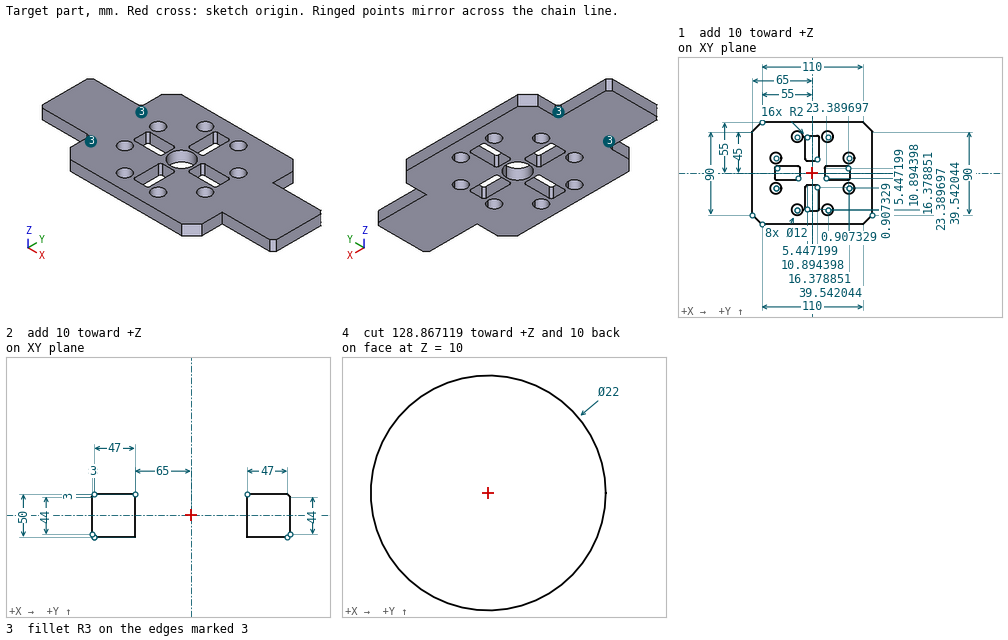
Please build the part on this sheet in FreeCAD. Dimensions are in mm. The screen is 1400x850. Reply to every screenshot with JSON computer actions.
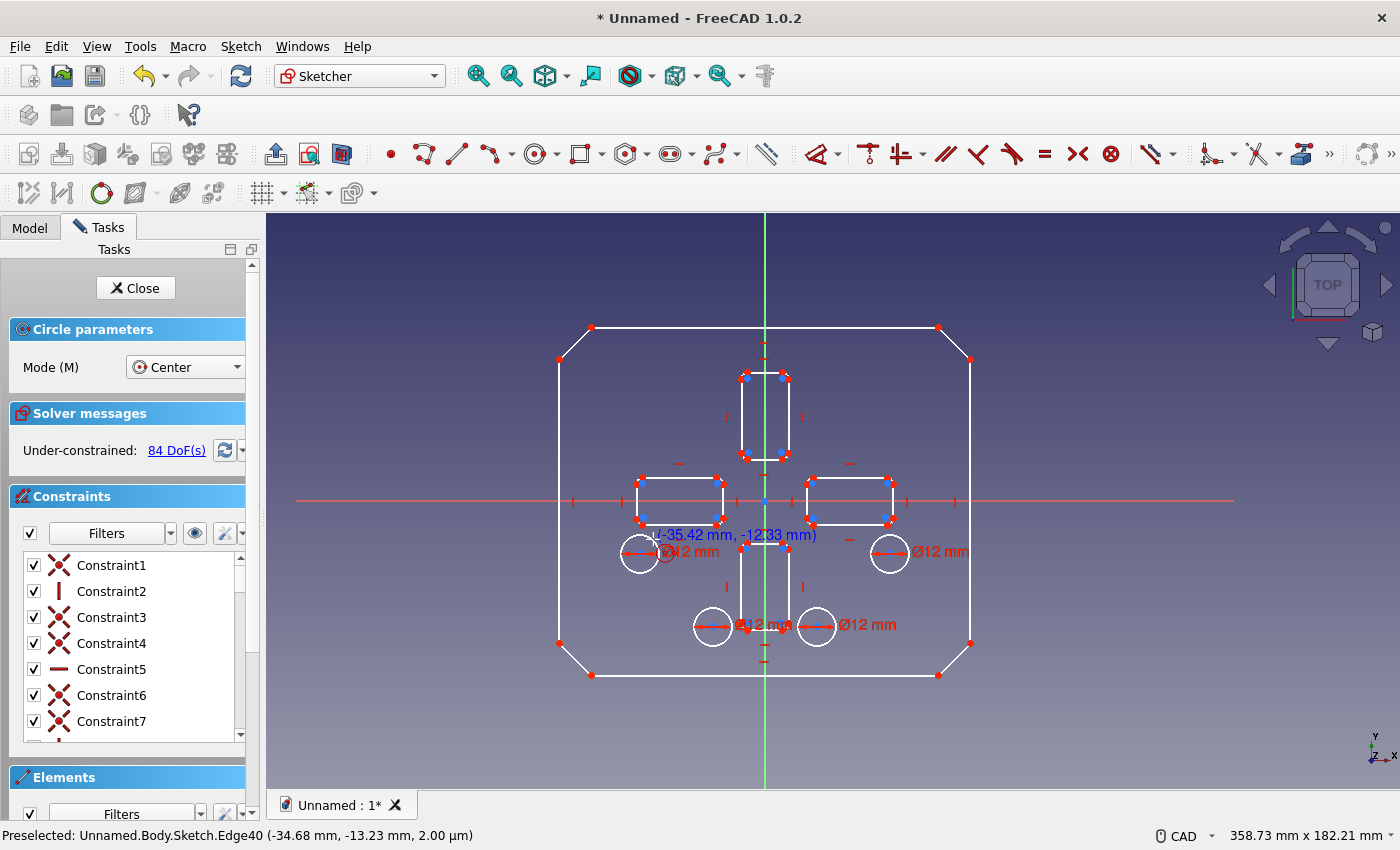
{"action": "left_click", "coordinate": [890, 449]}
{"action": "mouse_move", "coordinate": [903, 436]}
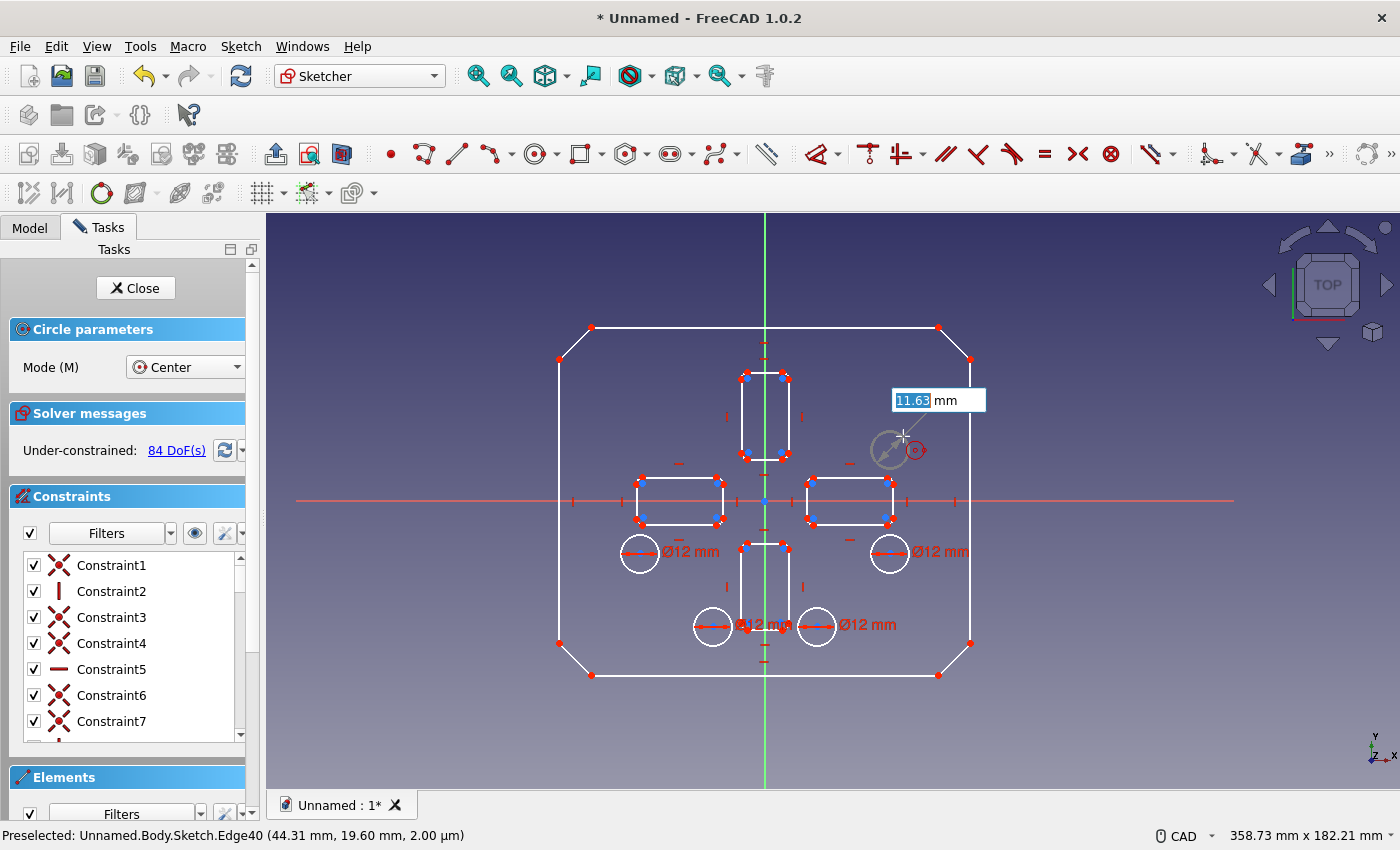
{"action": "type", "text": "12"}
{"action": "key", "text": "Return"}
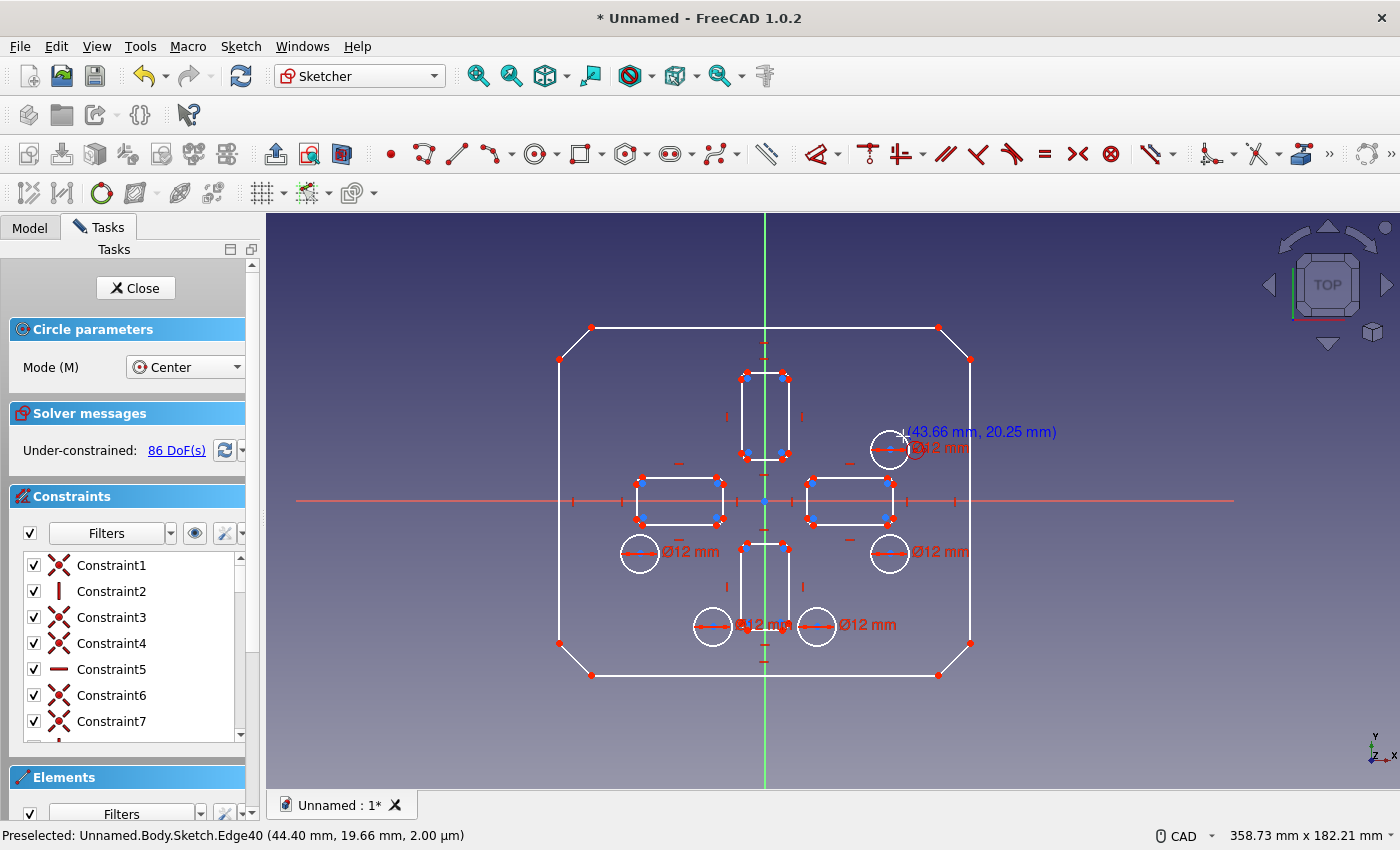
{"action": "left_click", "coordinate": [817, 376]}
{"action": "mouse_move", "coordinate": [830, 363]}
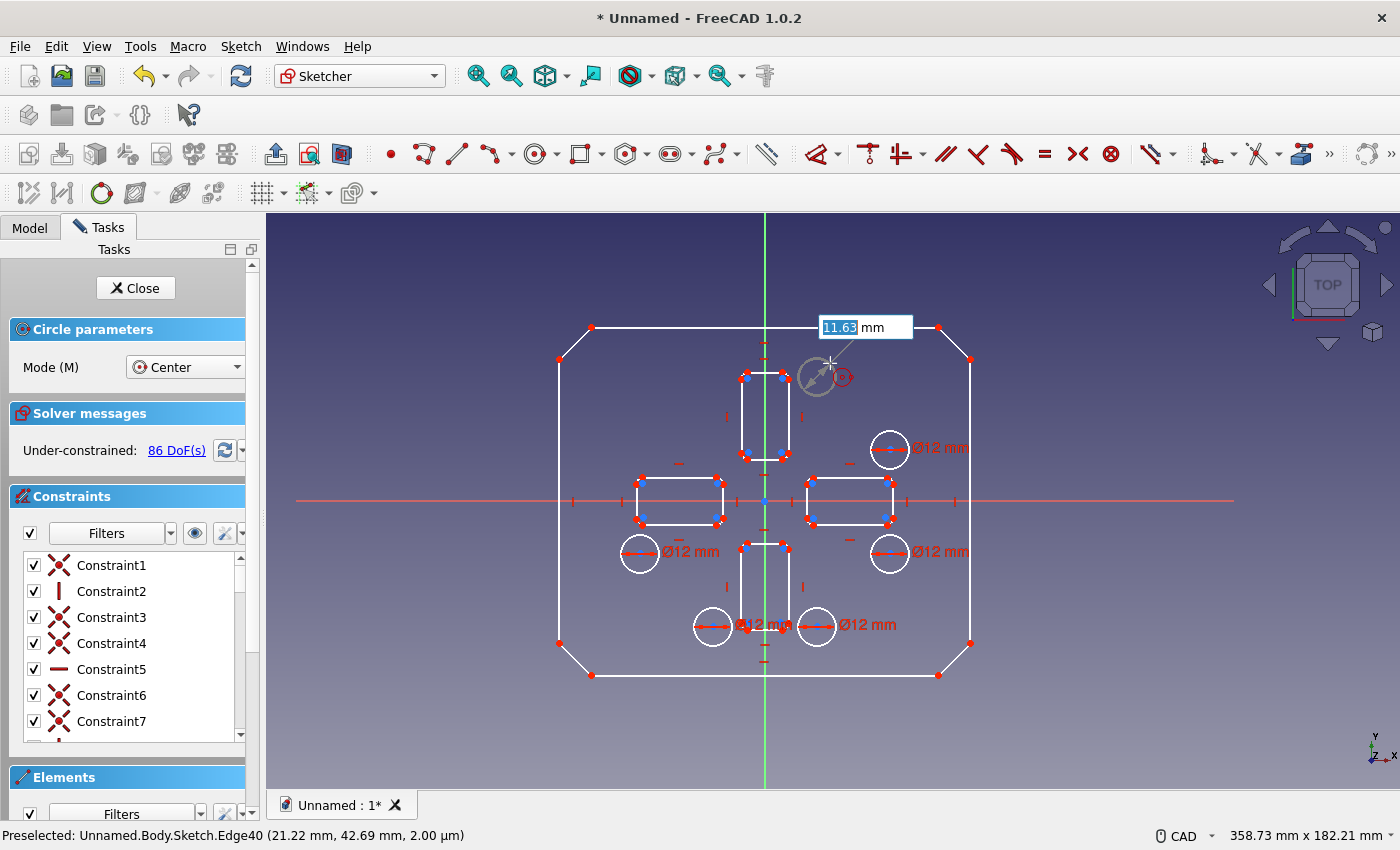
{"action": "type", "text": "12"}
{"action": "key", "text": "Return"}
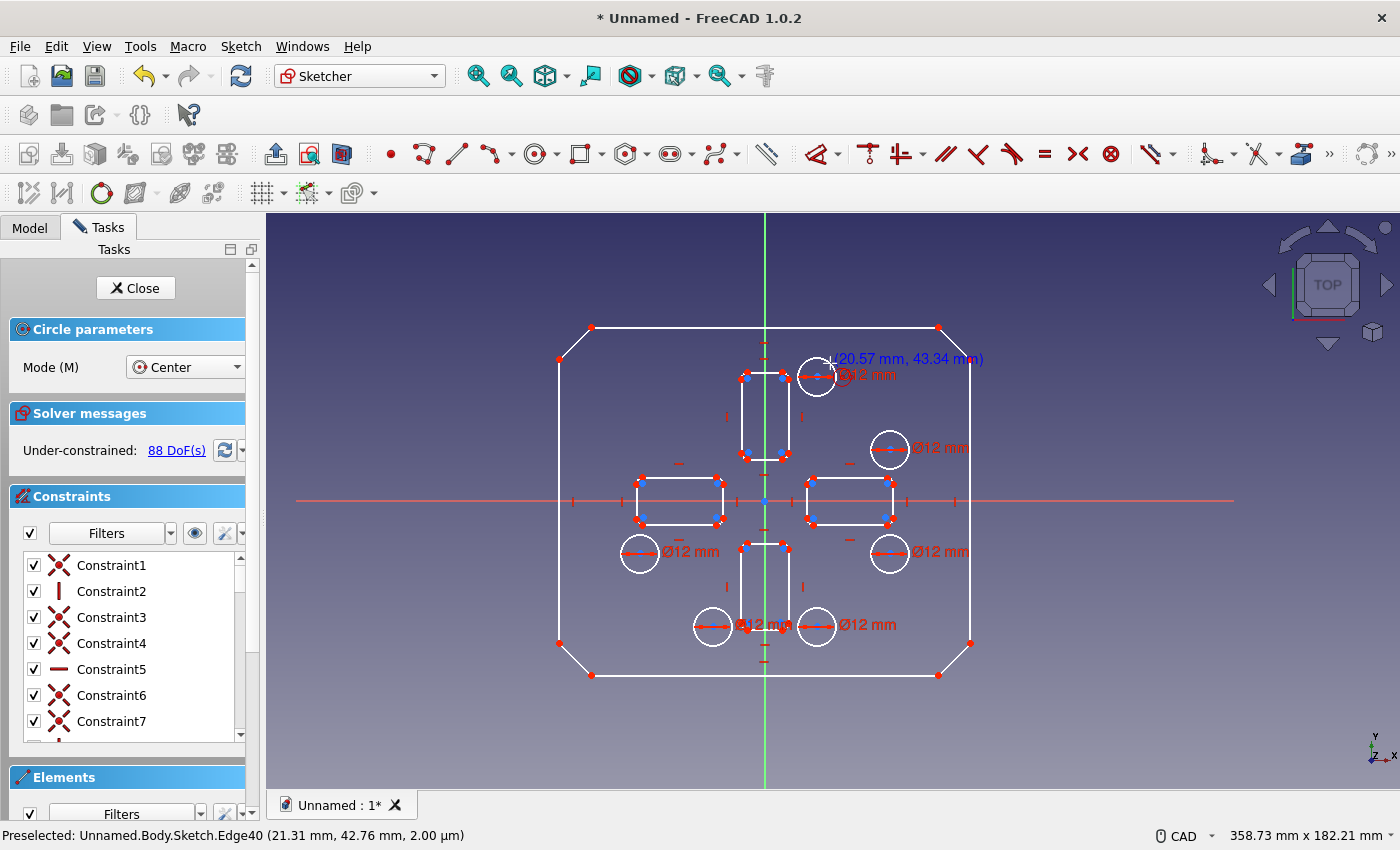
{"action": "left_click", "coordinate": [640, 449]}
{"action": "mouse_move", "coordinate": [653, 436]}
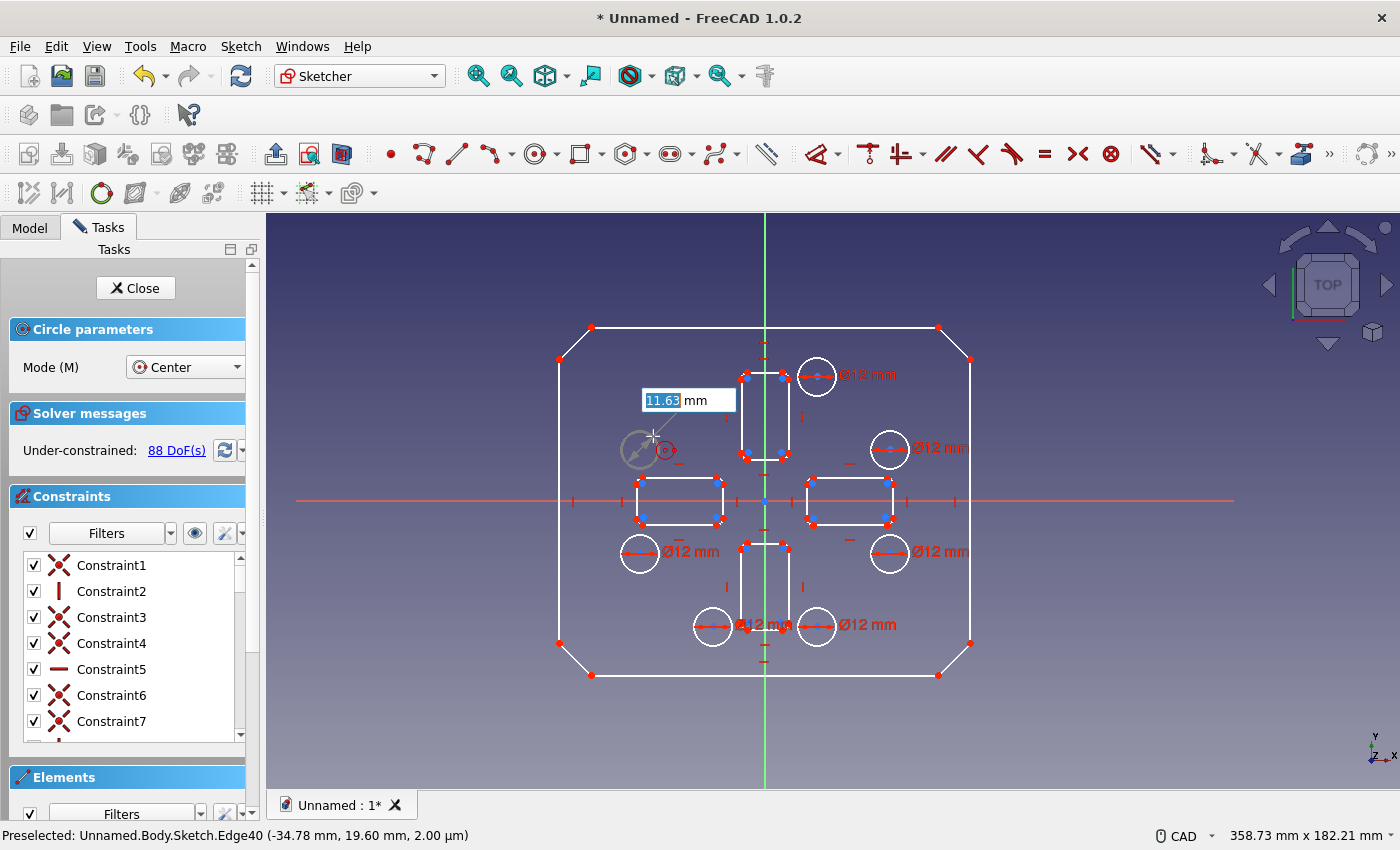
{"action": "type", "text": "12"}
{"action": "key", "text": "Return"}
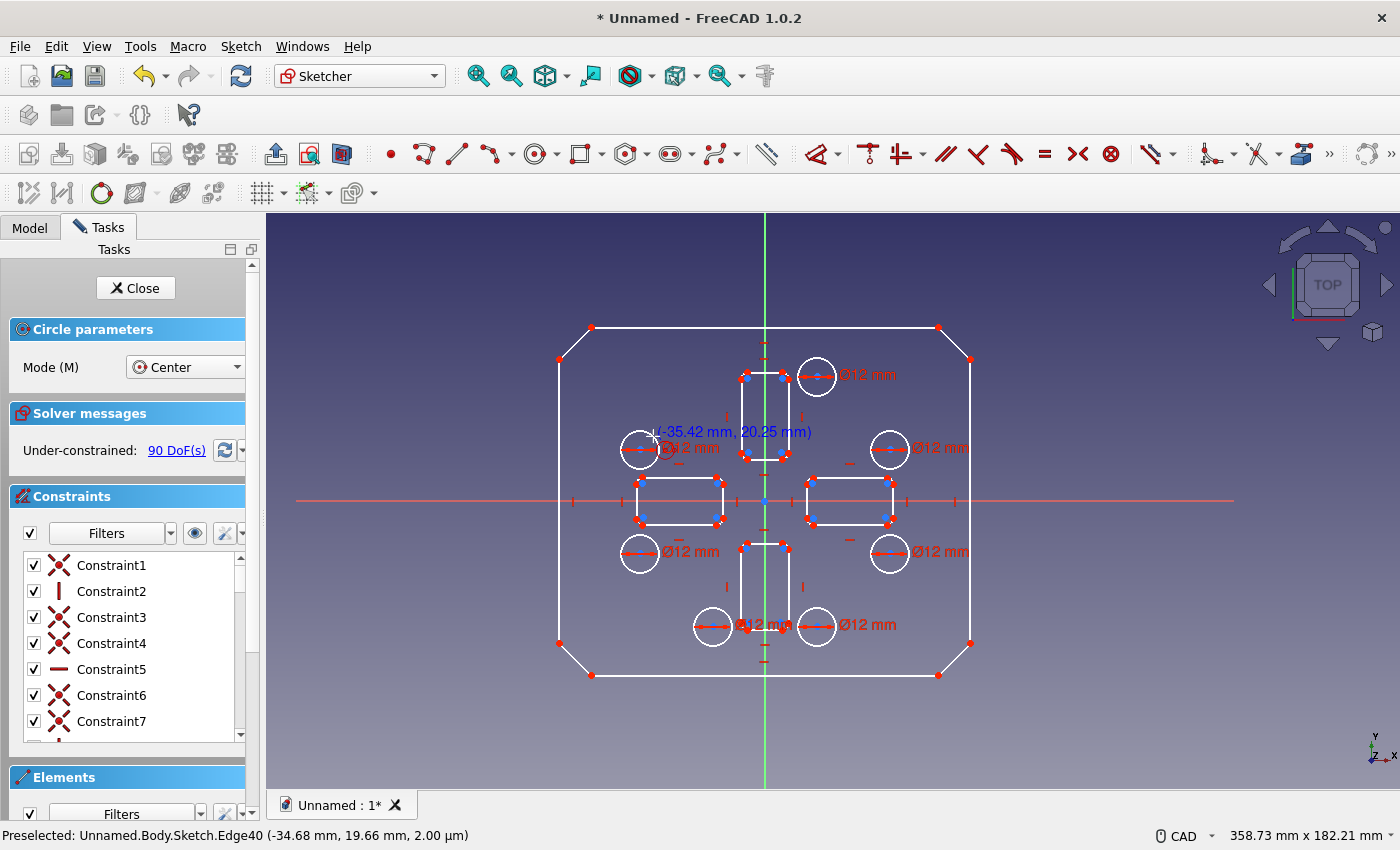
{"action": "left_click", "coordinate": [713, 376]}
{"action": "mouse_move", "coordinate": [727, 363]}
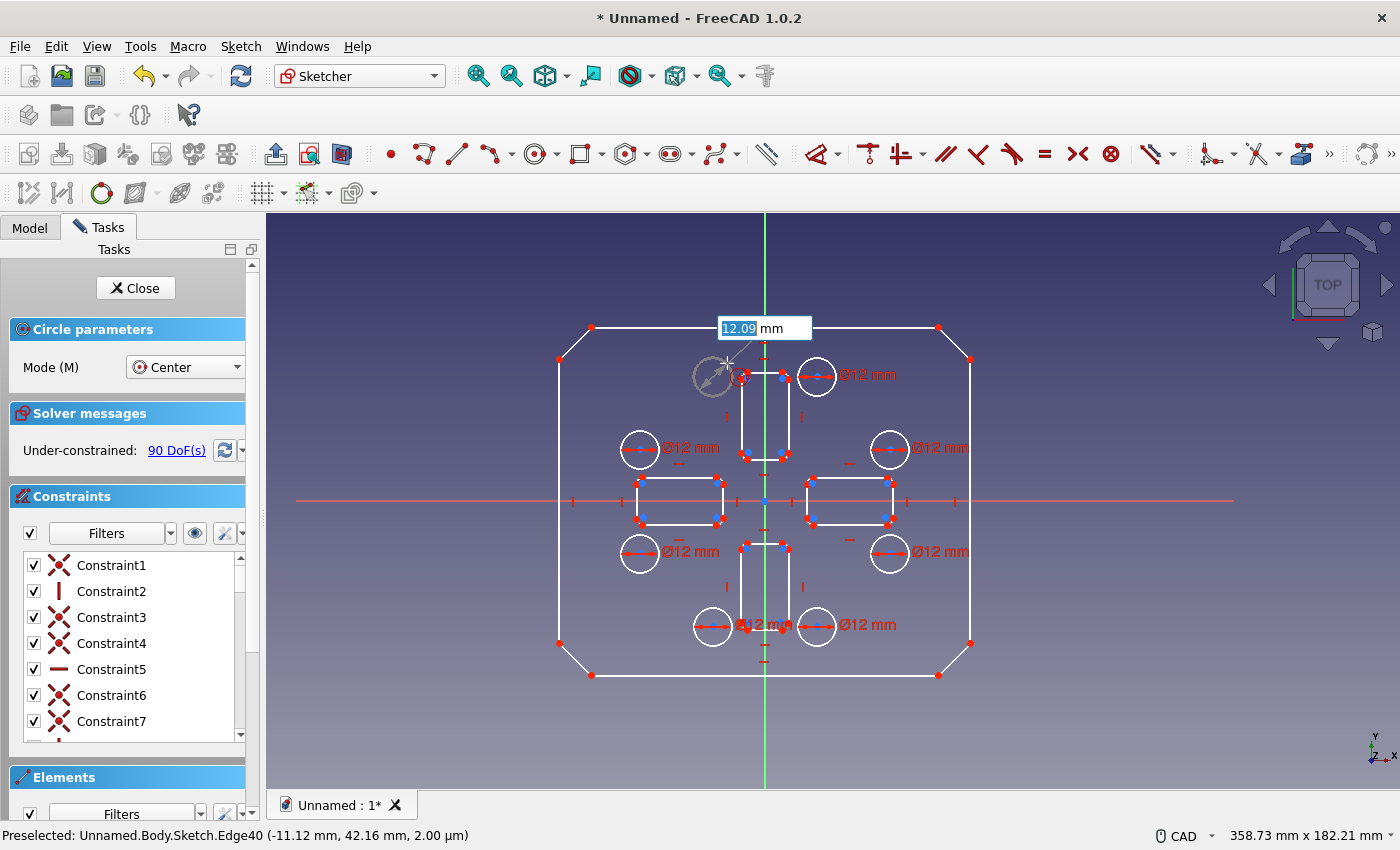
{"action": "type", "text": "12"}
{"action": "key", "text": "Return"}
{"action": "key", "text": "Escape"}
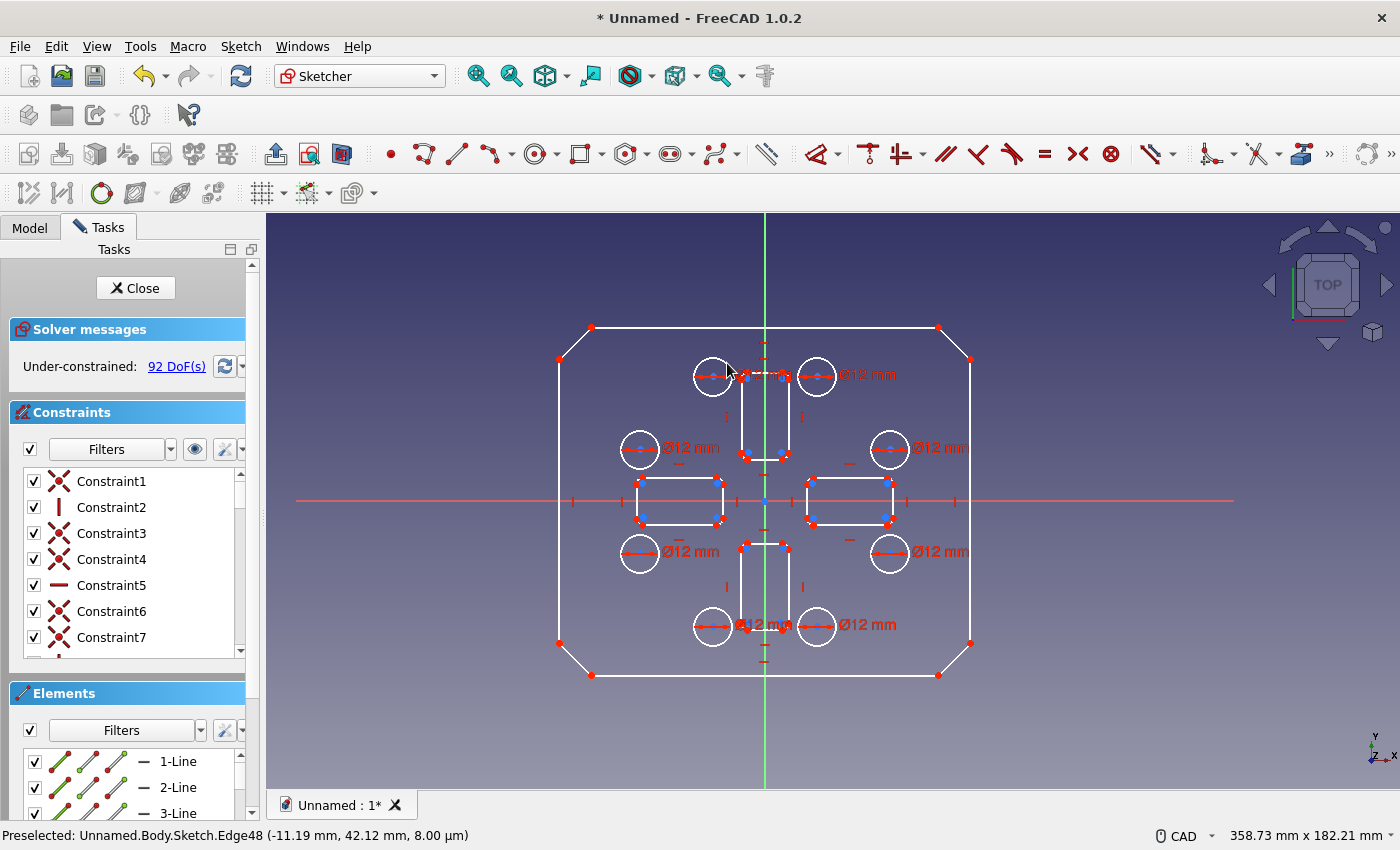
{"action": "left_click", "coordinate": [761, 544]}